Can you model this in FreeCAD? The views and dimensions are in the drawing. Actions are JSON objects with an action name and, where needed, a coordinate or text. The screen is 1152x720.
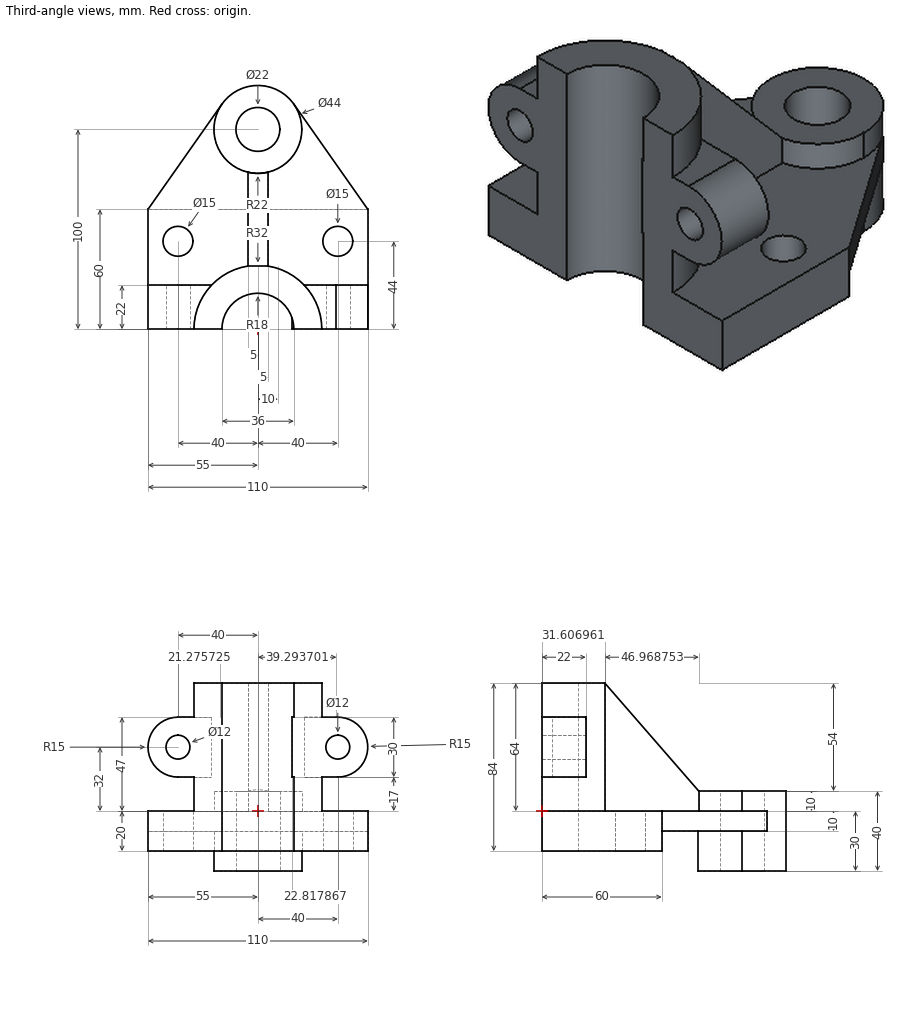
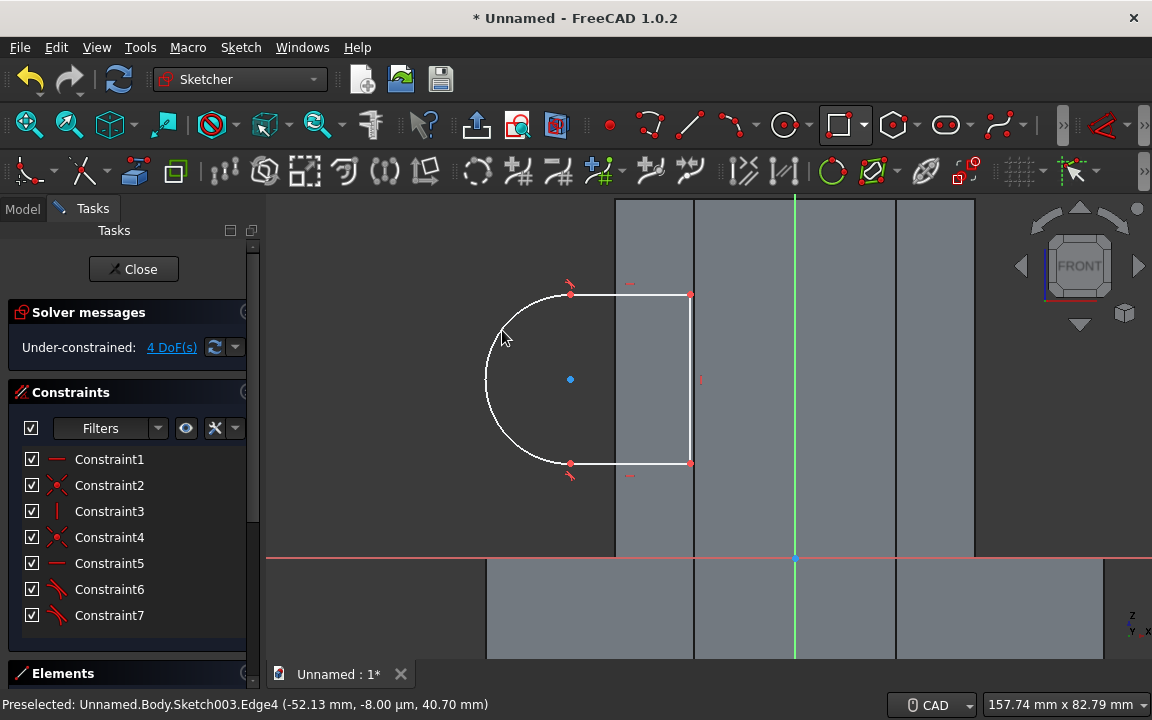
{"action": "left_click", "coordinate": [1102, 126]}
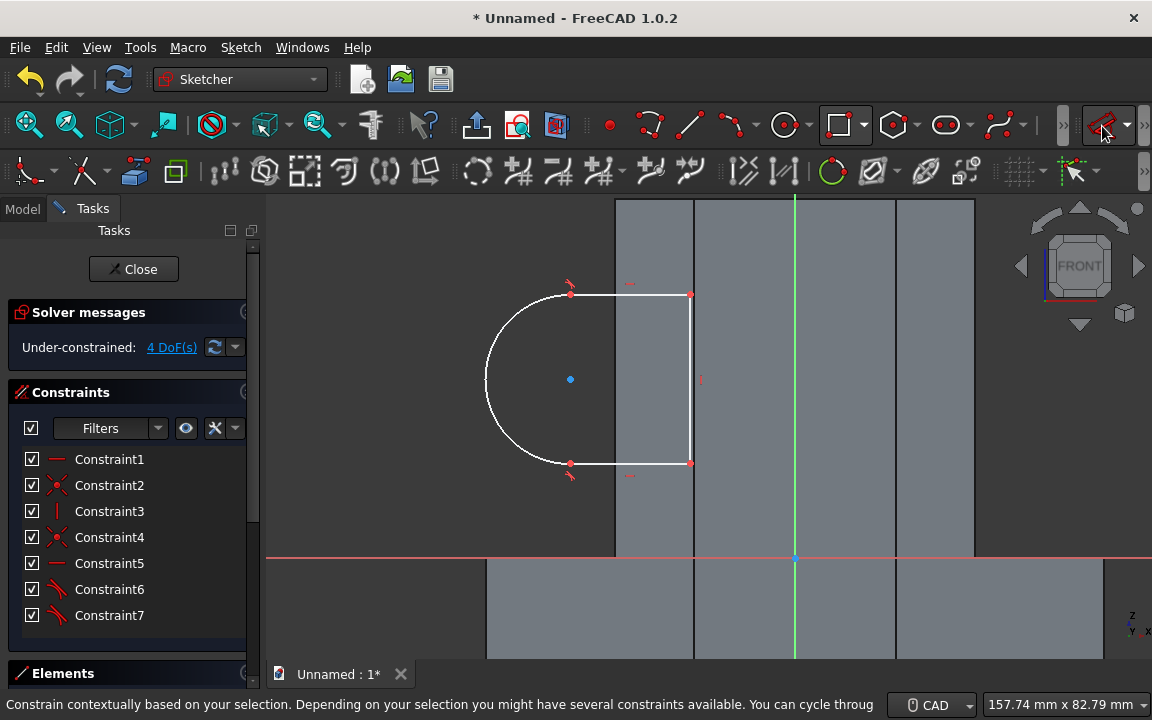
{"action": "left_click", "coordinate": [502, 330]}
{"action": "left_click", "coordinate": [476, 311]}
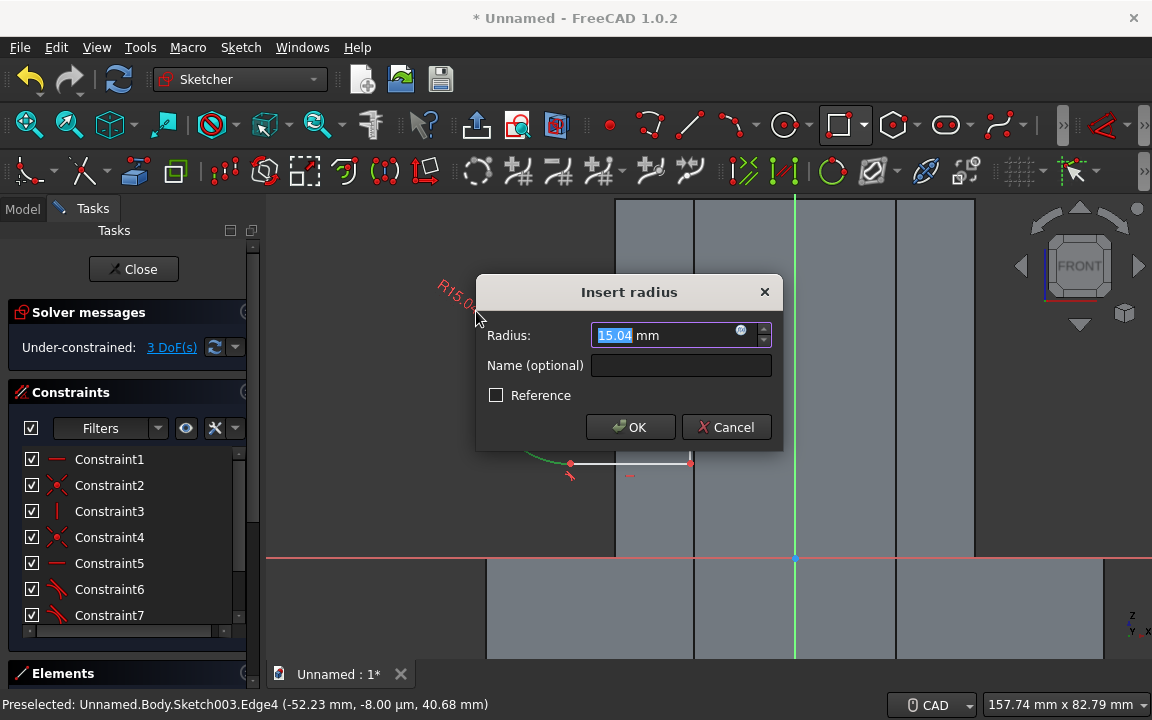
{"action": "type", "text": "15"}
{"action": "key", "text": "Return"}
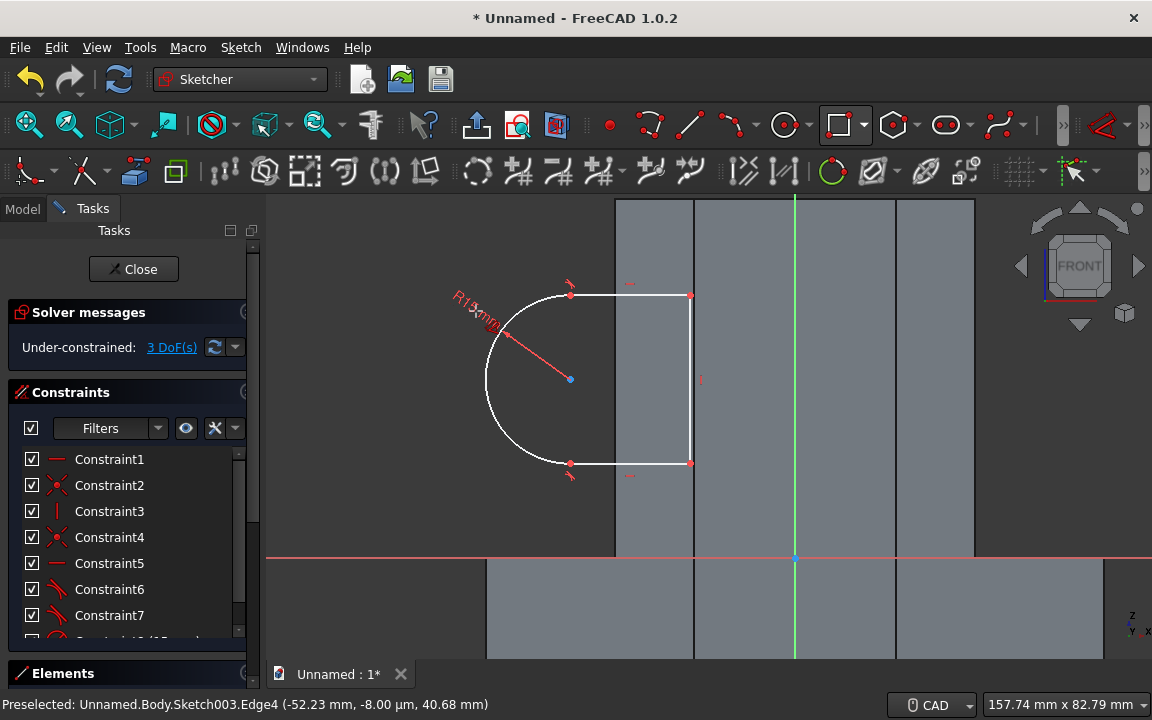
{"action": "left_click", "coordinate": [570, 295]}
{"action": "left_click", "coordinate": [683, 592]}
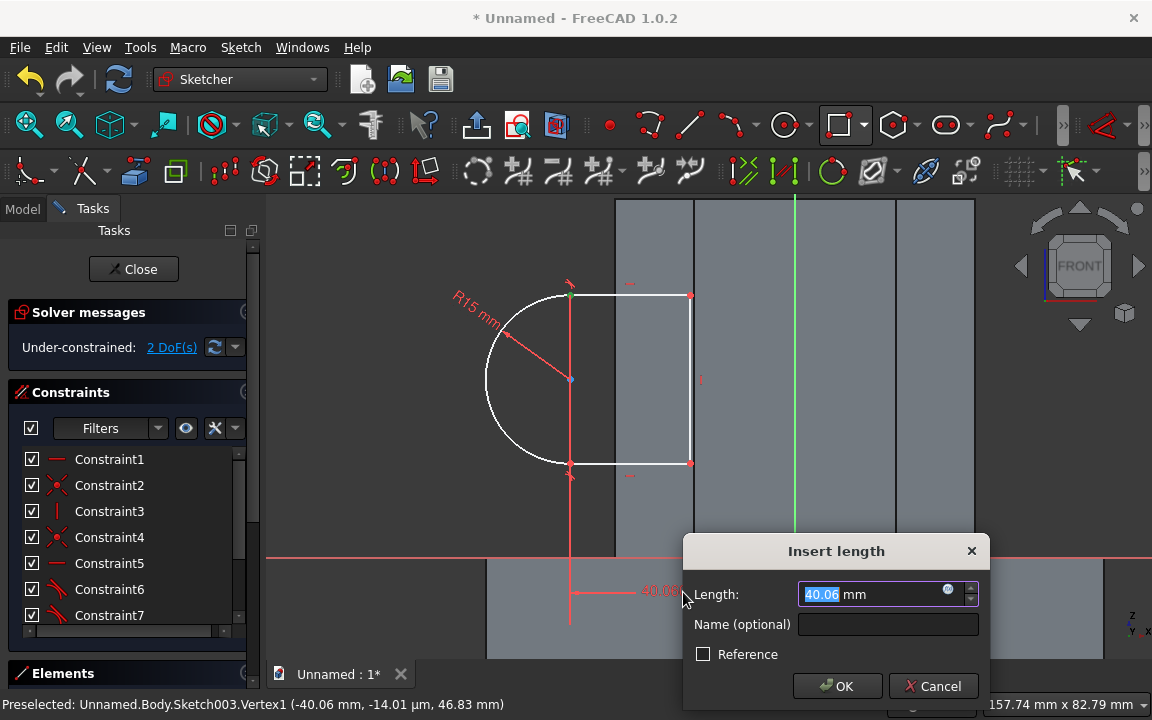
{"action": "type", "text": "40"}
{"action": "key", "text": "Return"}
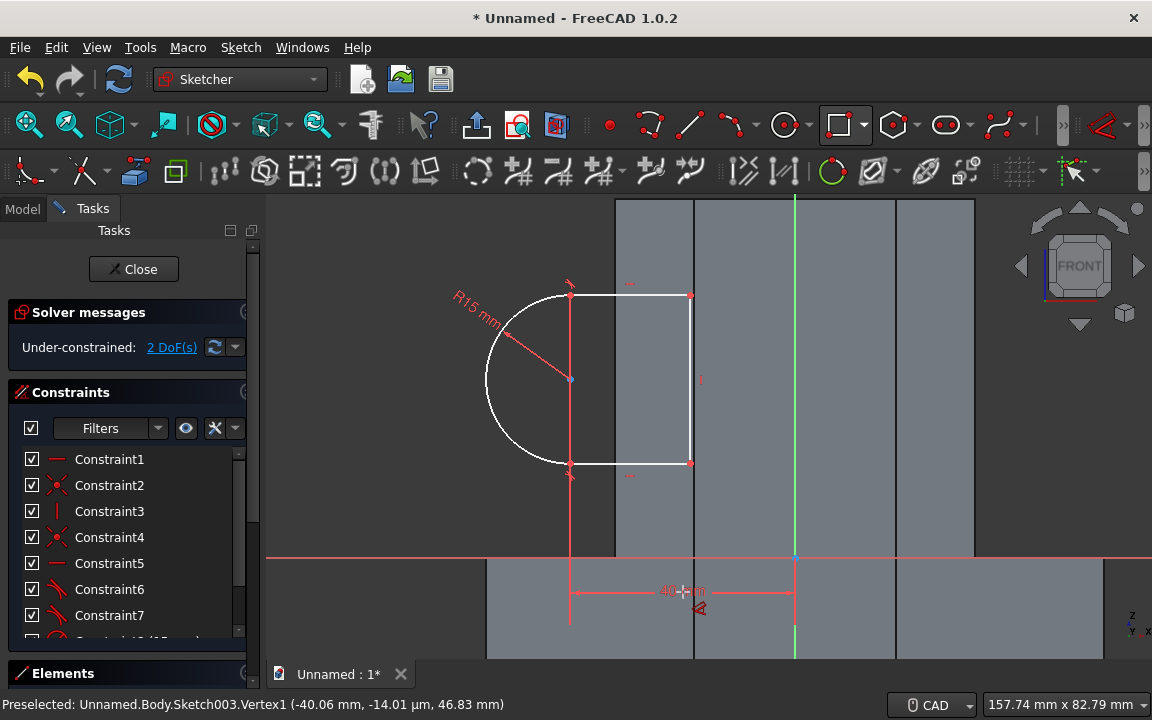
{"action": "left_click", "coordinate": [570, 295]}
{"action": "left_click", "coordinate": [829, 427]}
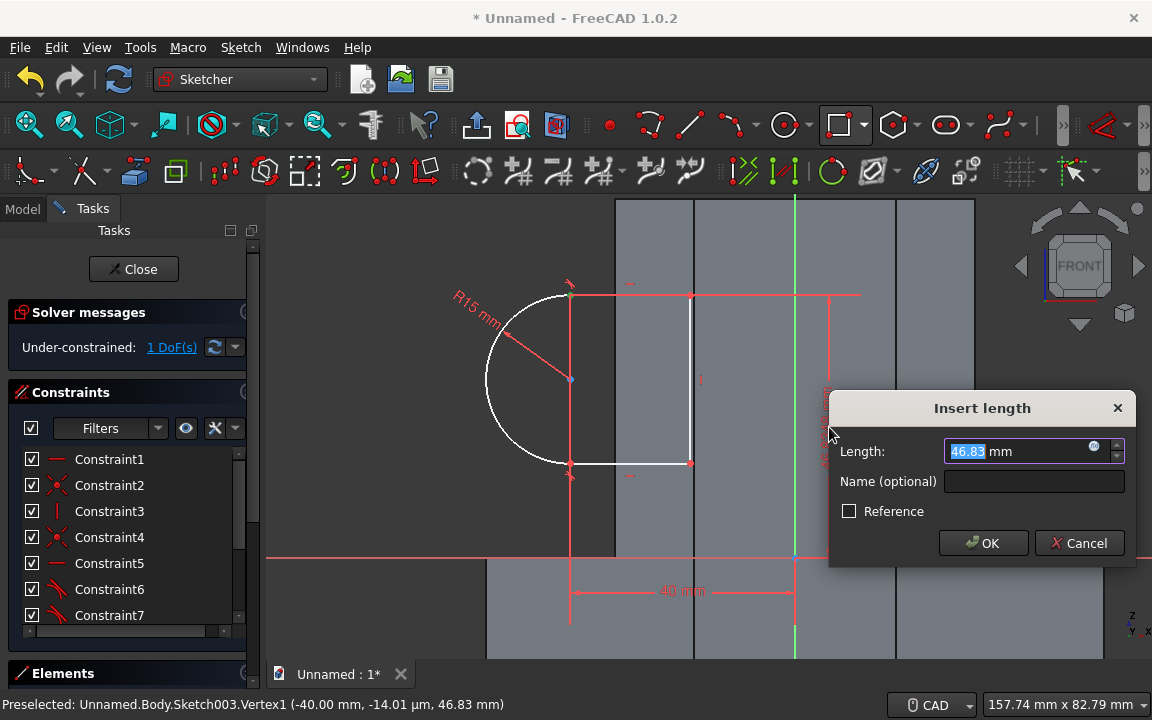
{"action": "type", "text": "47"}
{"action": "key", "text": "Return"}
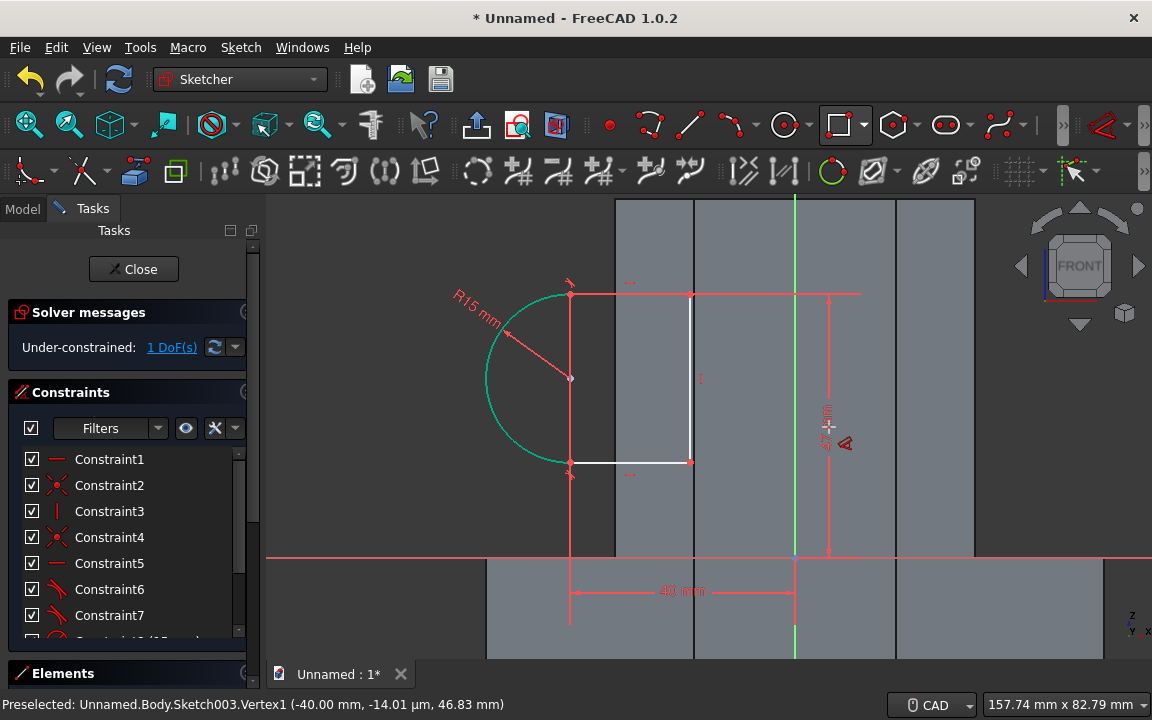
{"action": "left_click", "coordinate": [606, 294]}
{"action": "left_click", "coordinate": [630, 260]}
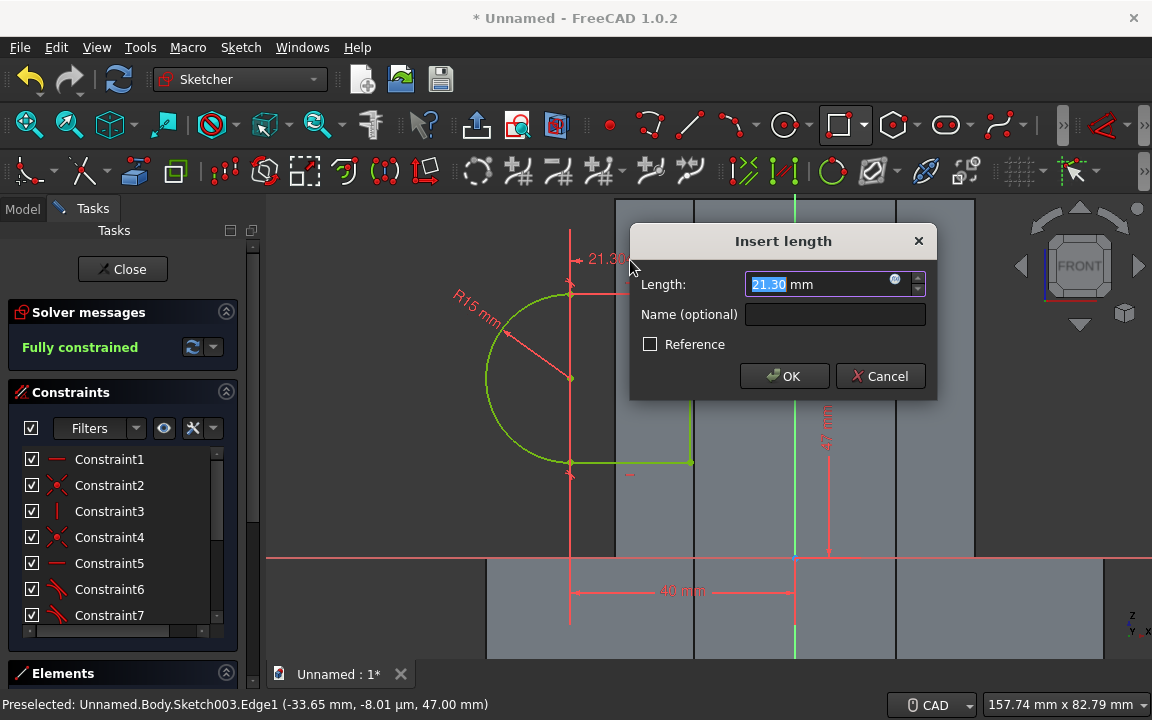
{"action": "type", "text": "21.275725"}
{"action": "key", "text": "Return"}
{"action": "key", "text": "Escape"}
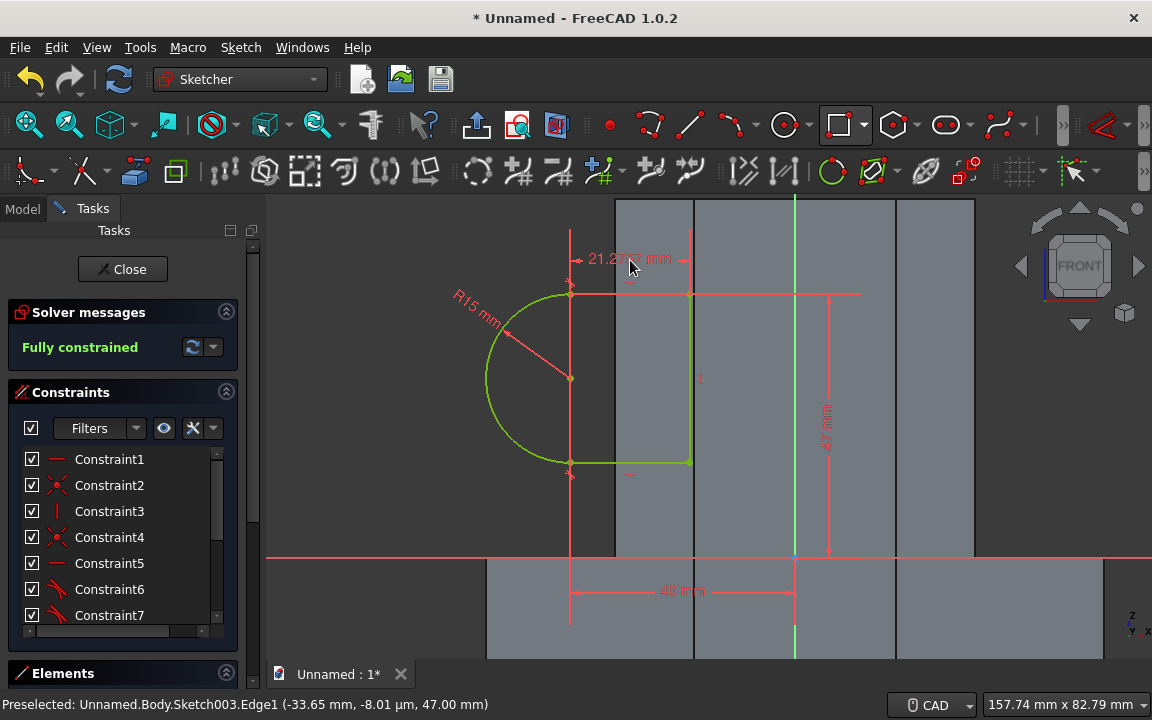
{"action": "left_click", "coordinate": [123, 269]}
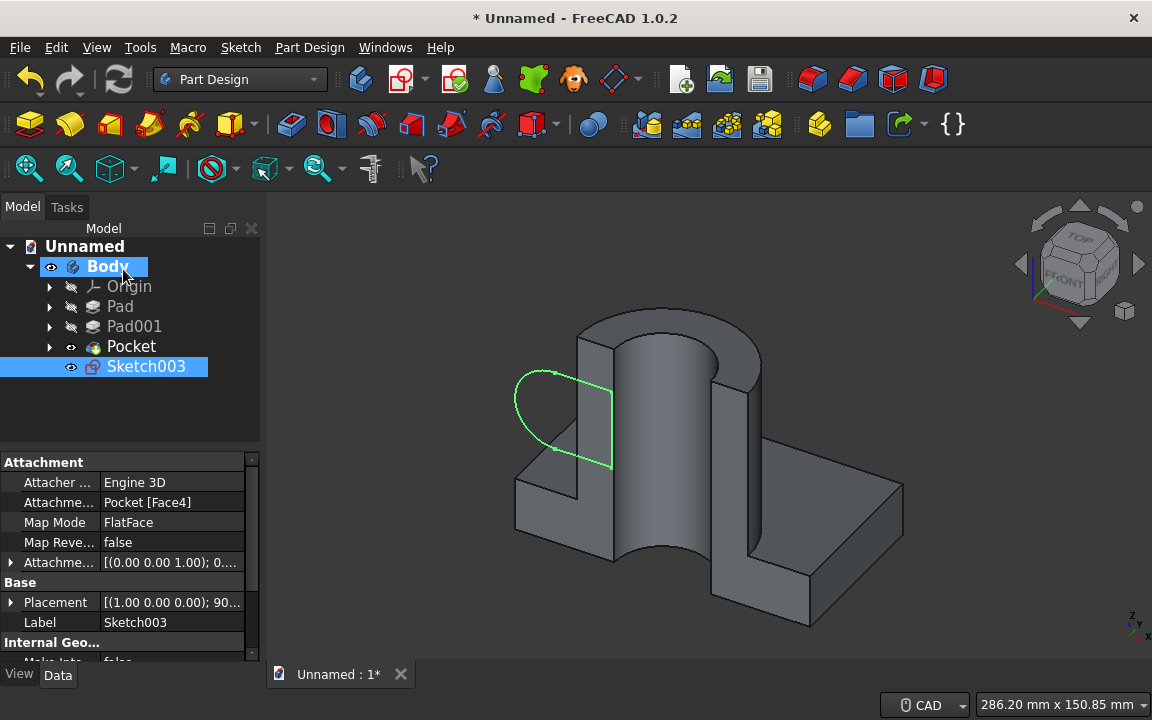
{"action": "left_click", "coordinate": [30, 124]}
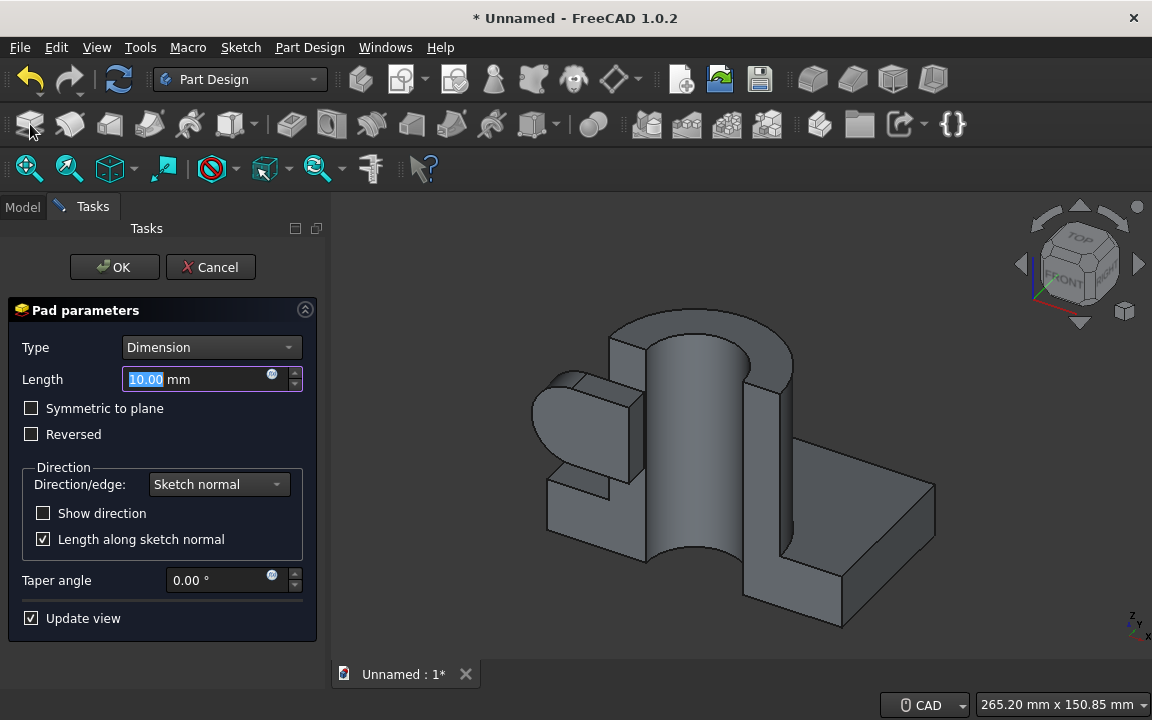
{"action": "type", "text": "22"}
{"action": "key", "text": "Tab"}